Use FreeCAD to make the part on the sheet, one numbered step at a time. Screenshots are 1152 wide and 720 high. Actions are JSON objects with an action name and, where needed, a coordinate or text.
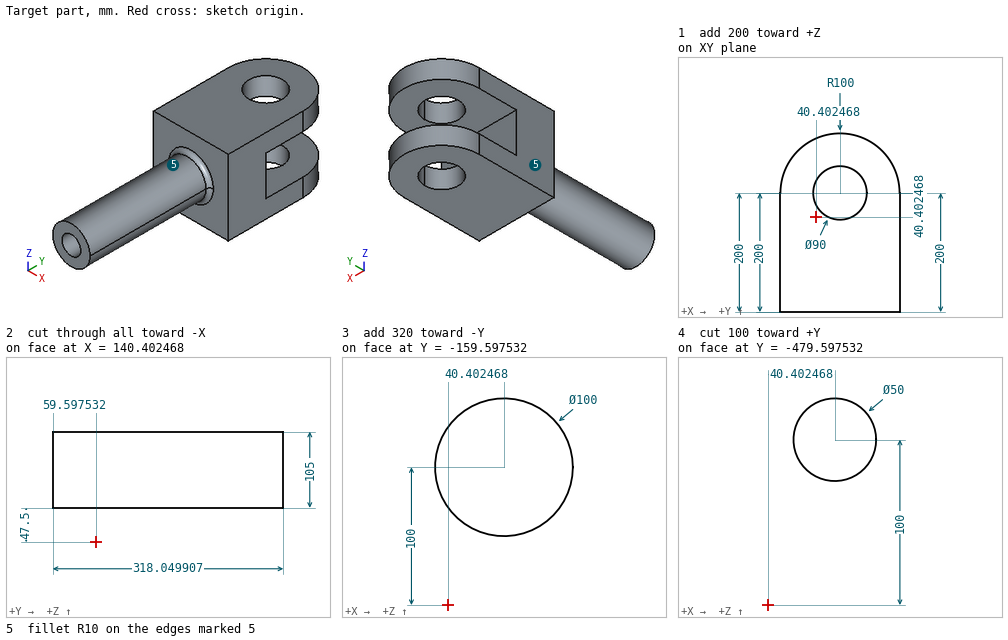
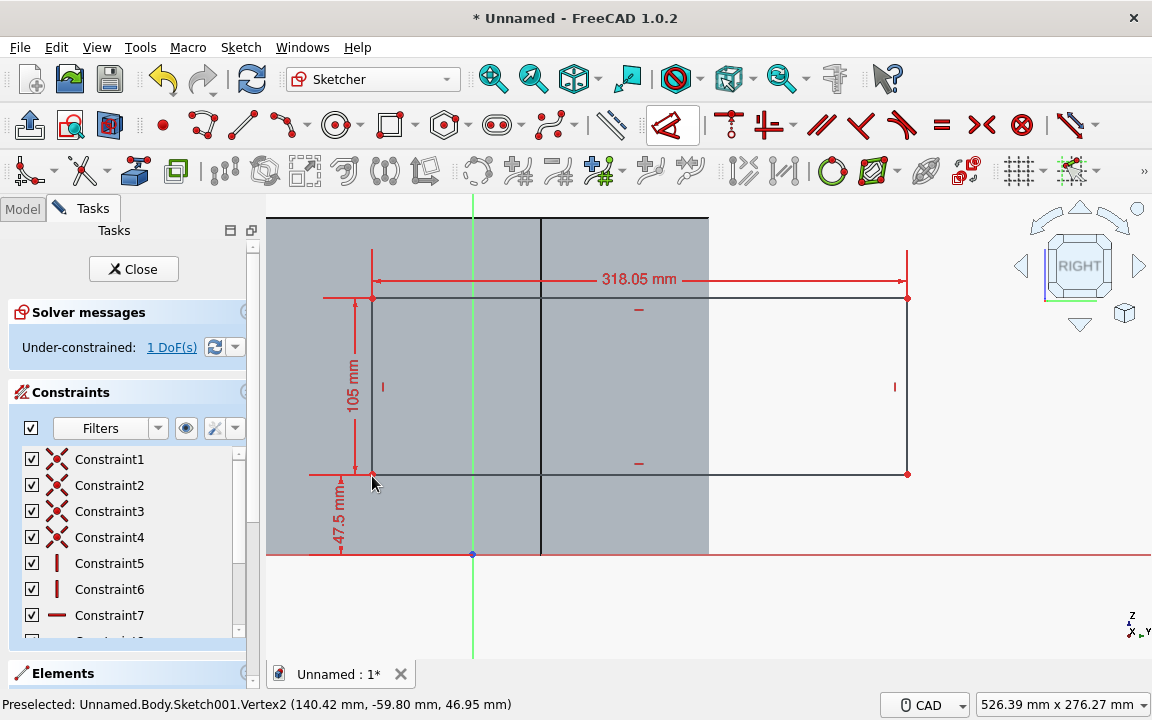
{"action": "left_click", "coordinate": [372, 298]}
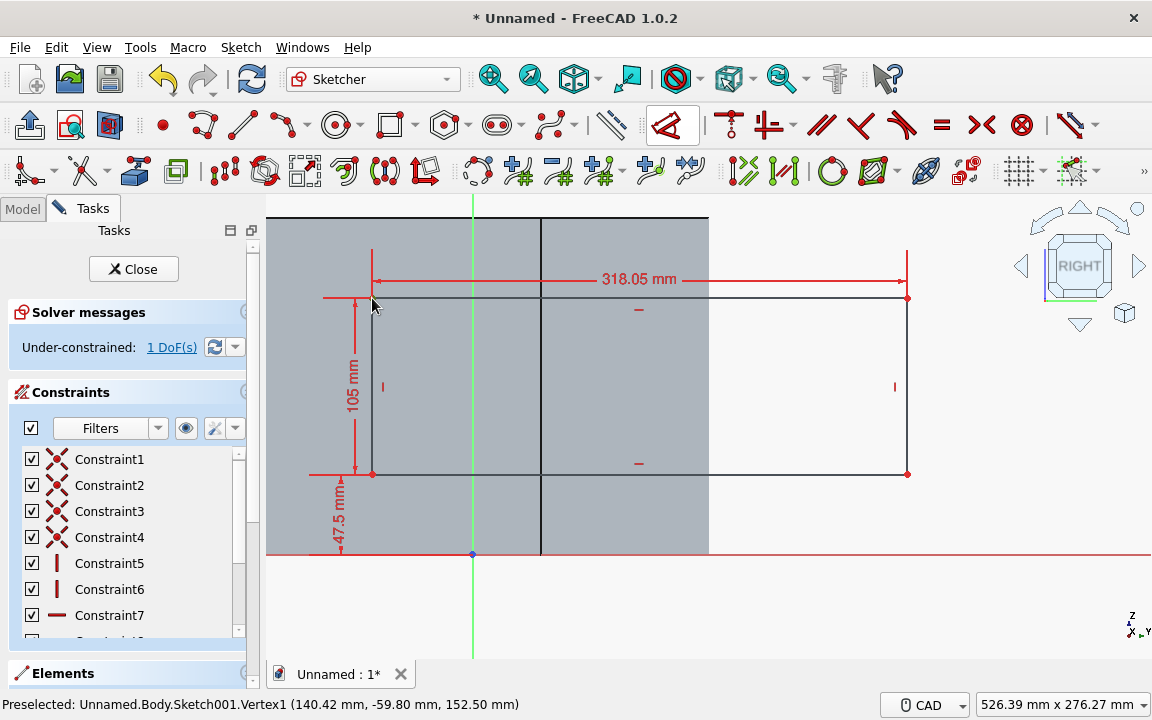
{"action": "key", "text": "l"}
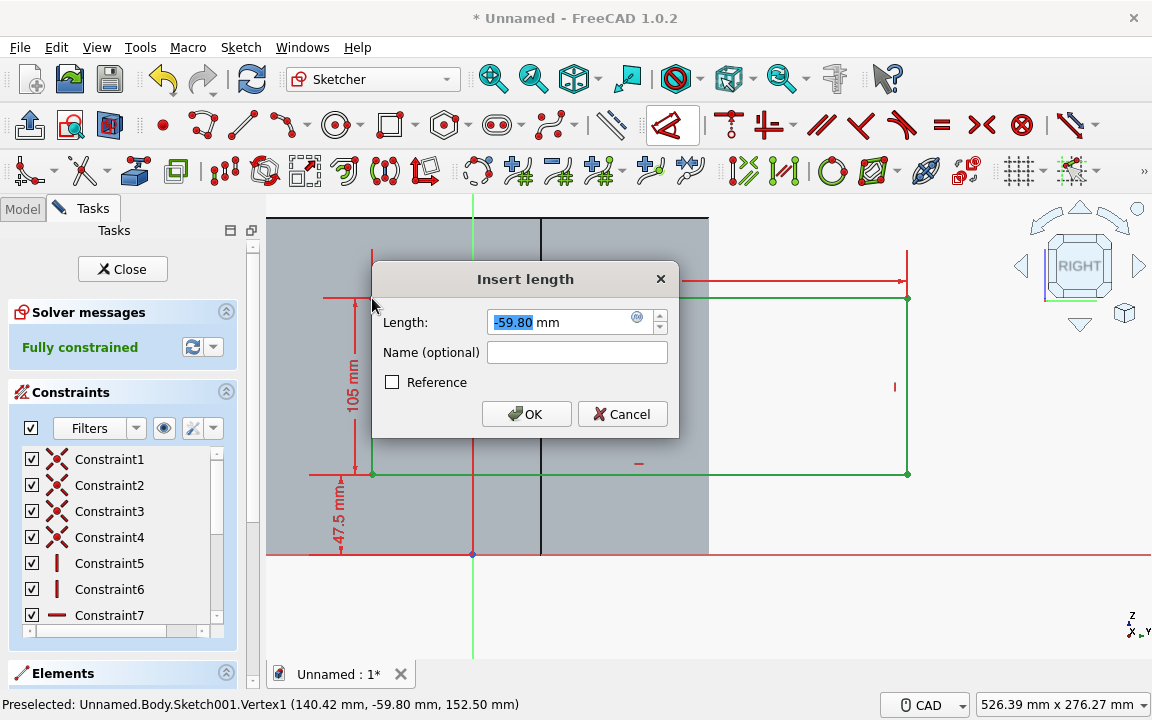
{"action": "type", "text": "-59.597532"}
{"action": "key", "text": "Return"}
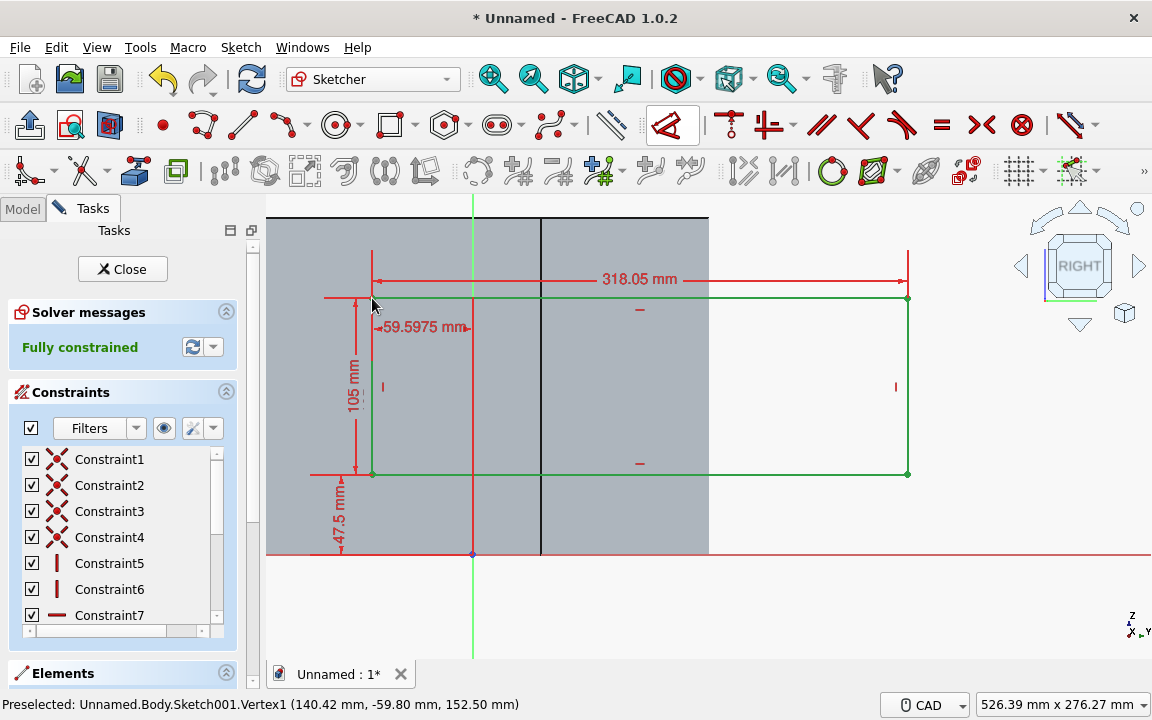
{"action": "left_click", "coordinate": [123, 269]}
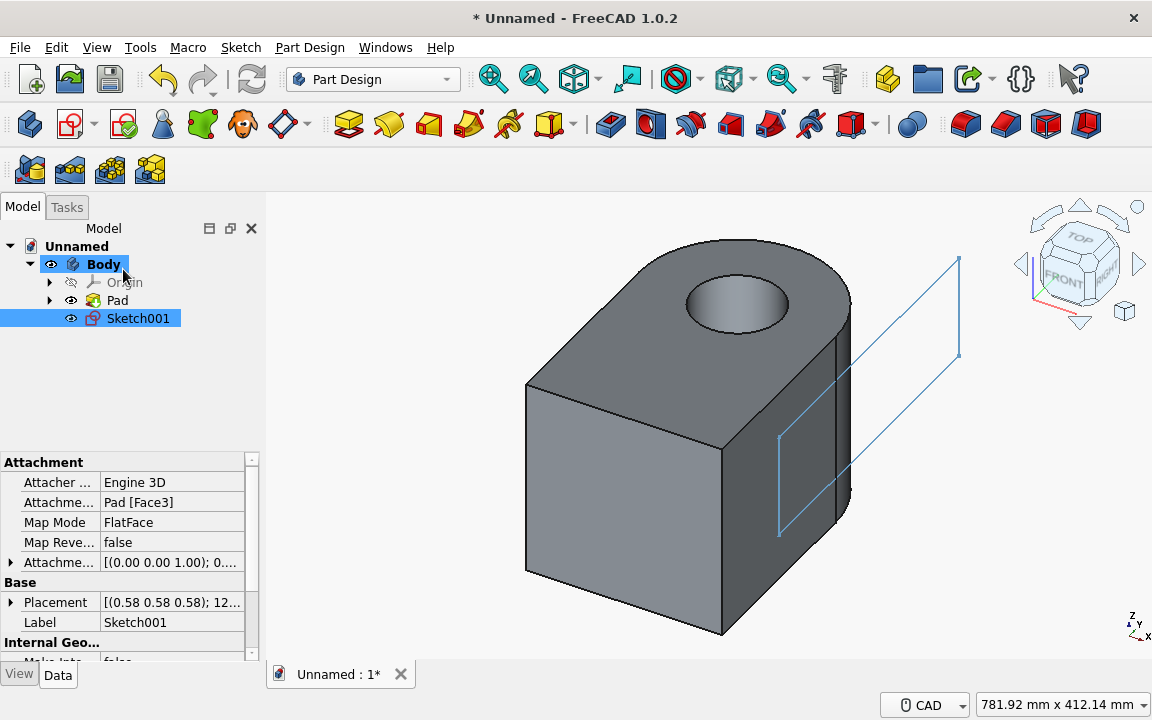
{"action": "left_click", "coordinate": [612, 124]}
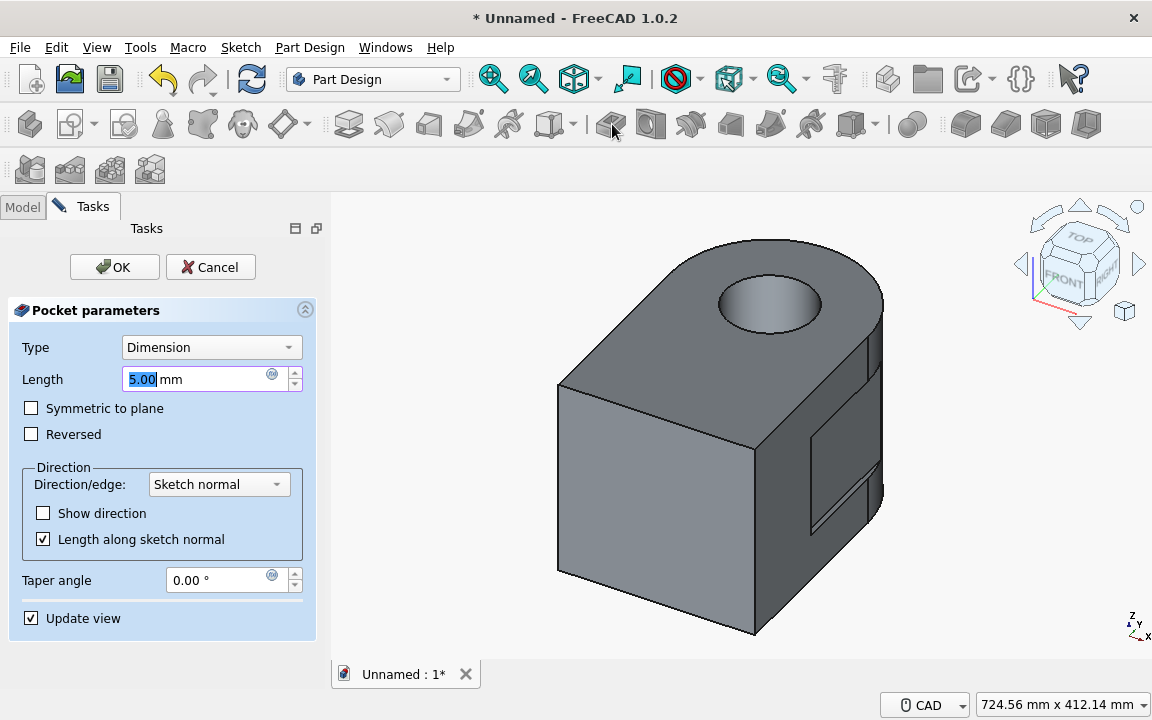
{"action": "left_click", "coordinate": [212, 348]}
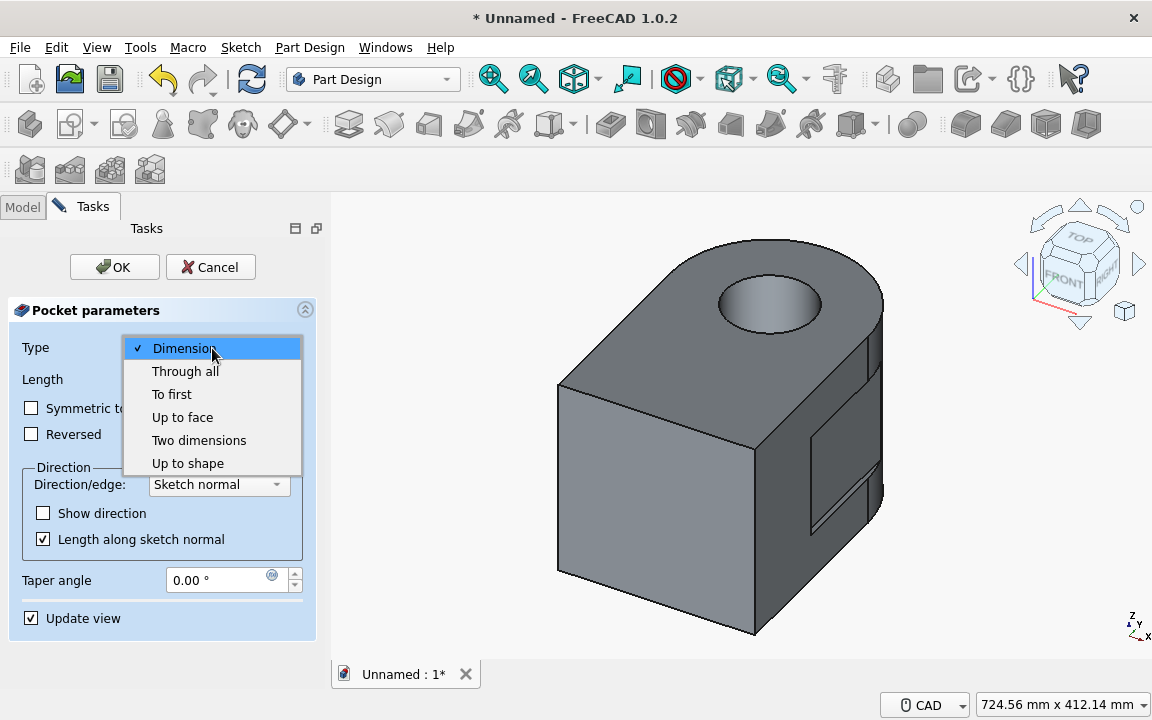
{"action": "left_click", "coordinate": [212, 372]}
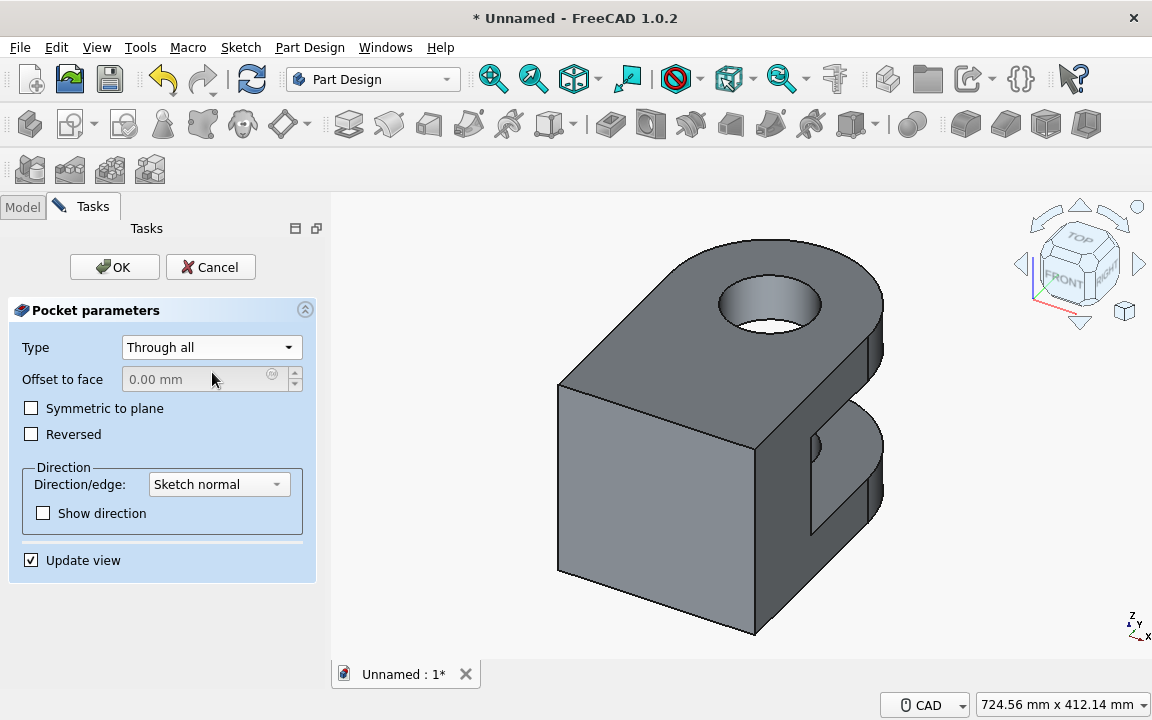
{"action": "left_click", "coordinate": [115, 267]}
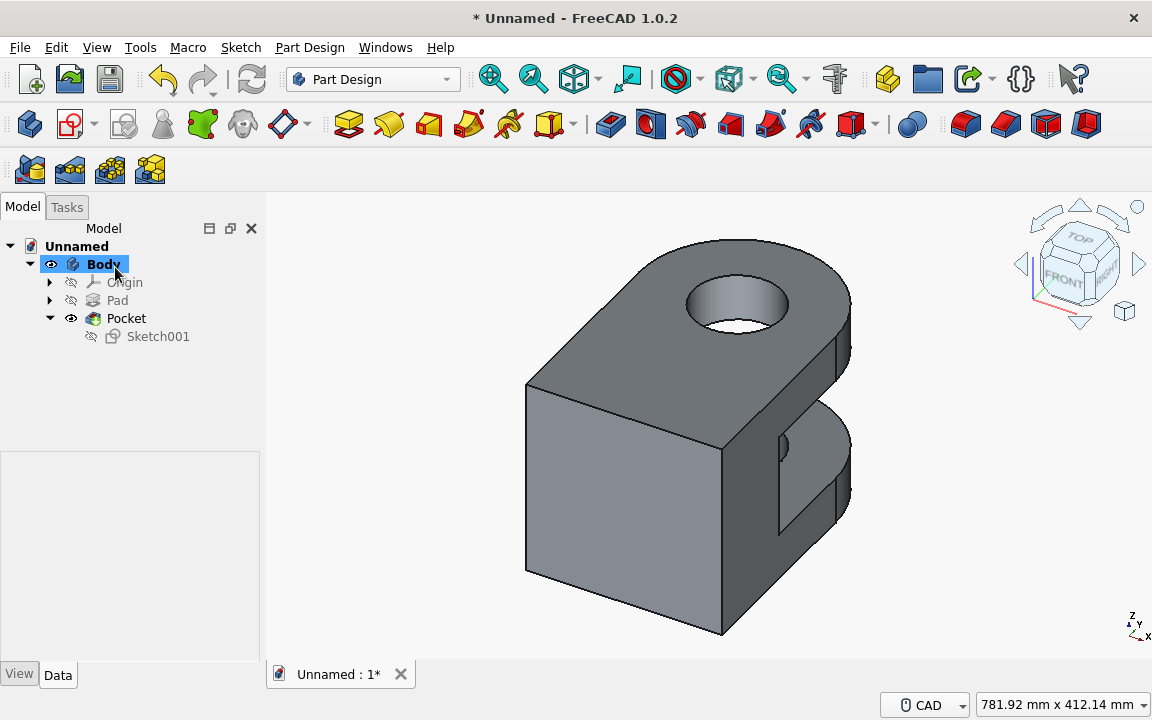
{"action": "left_click", "coordinate": [624, 509]}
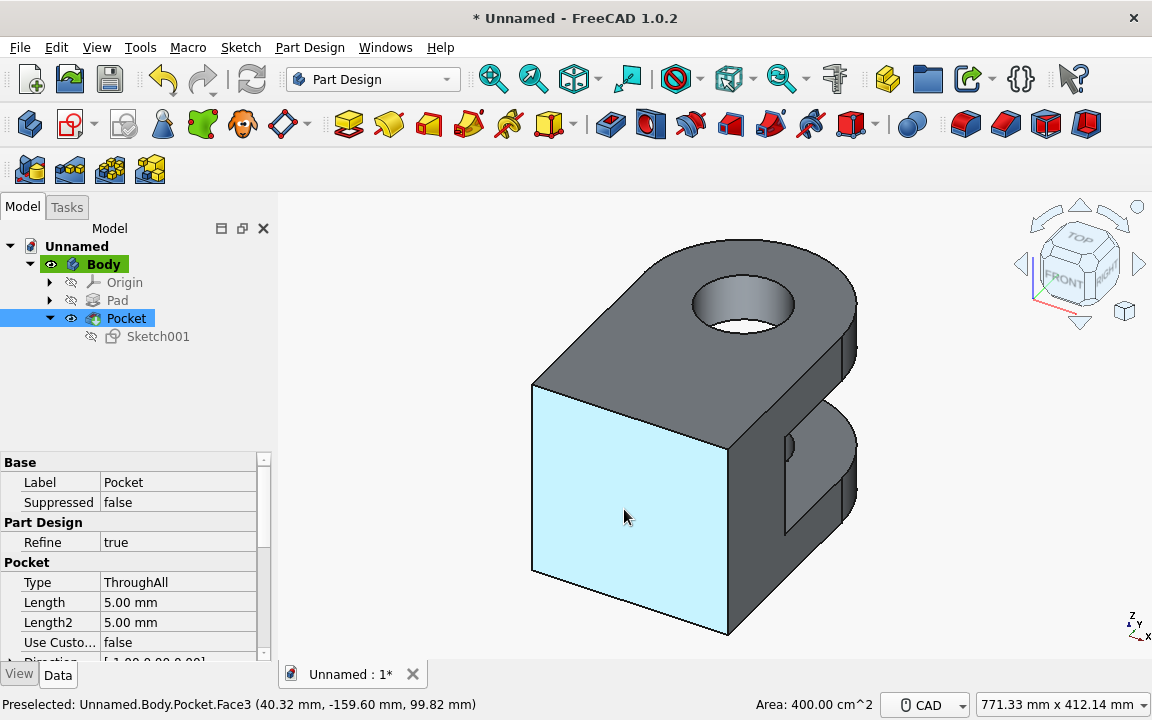
{"action": "left_click", "coordinate": [70, 124]}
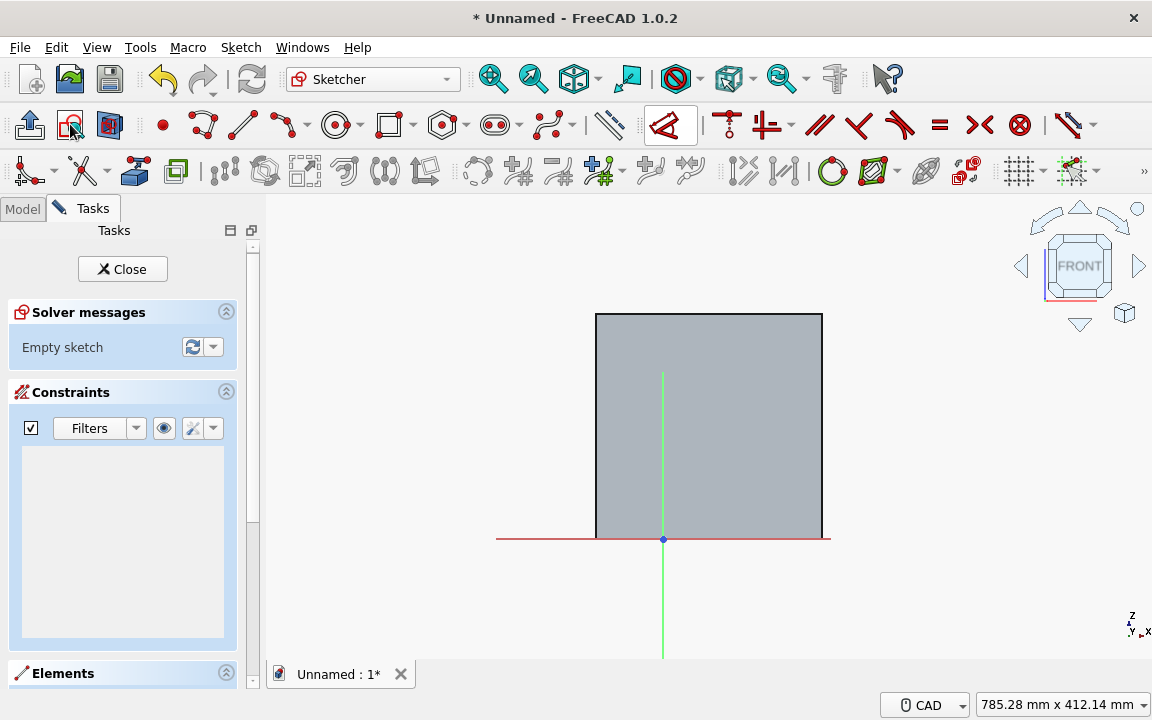
{"action": "scroll", "coordinate": [792, 489], "scroll_direction": "up", "scroll_amount": 3}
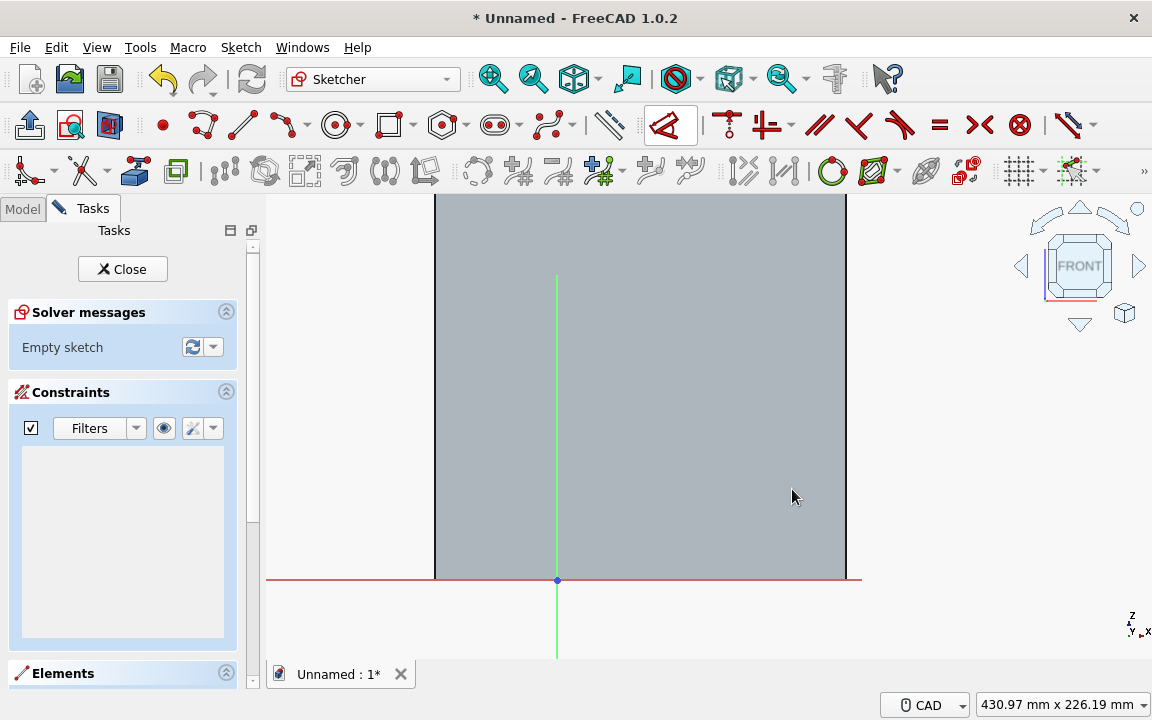
{"action": "key", "text": "g c"}